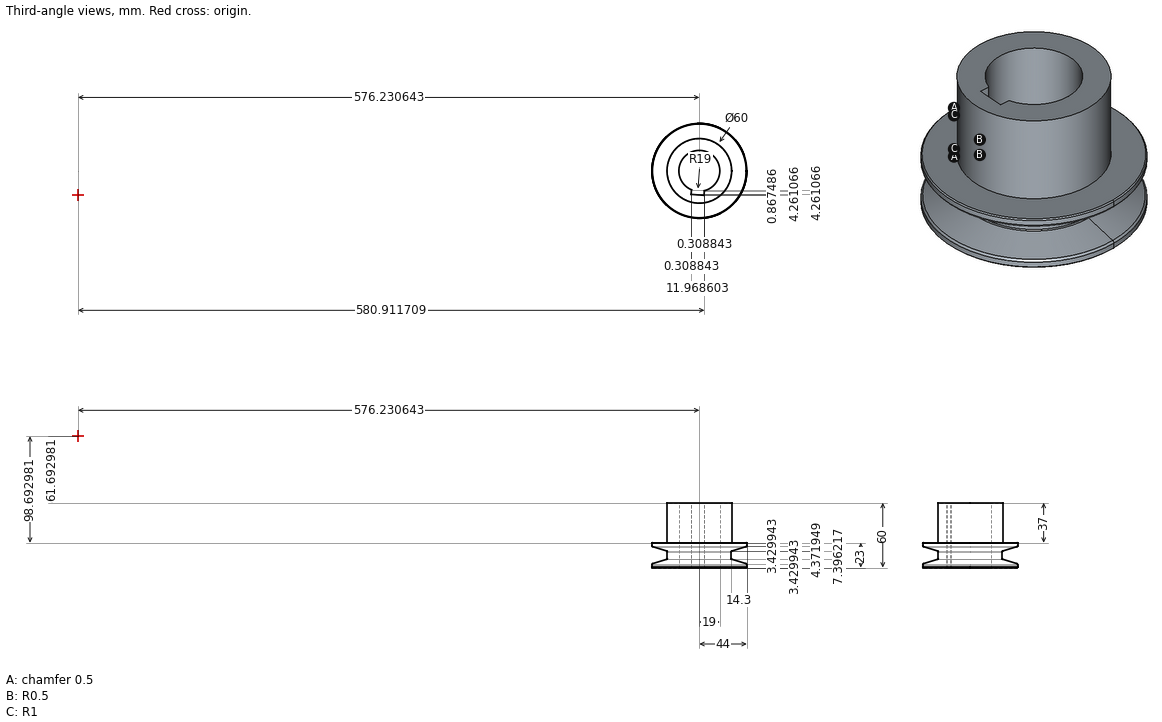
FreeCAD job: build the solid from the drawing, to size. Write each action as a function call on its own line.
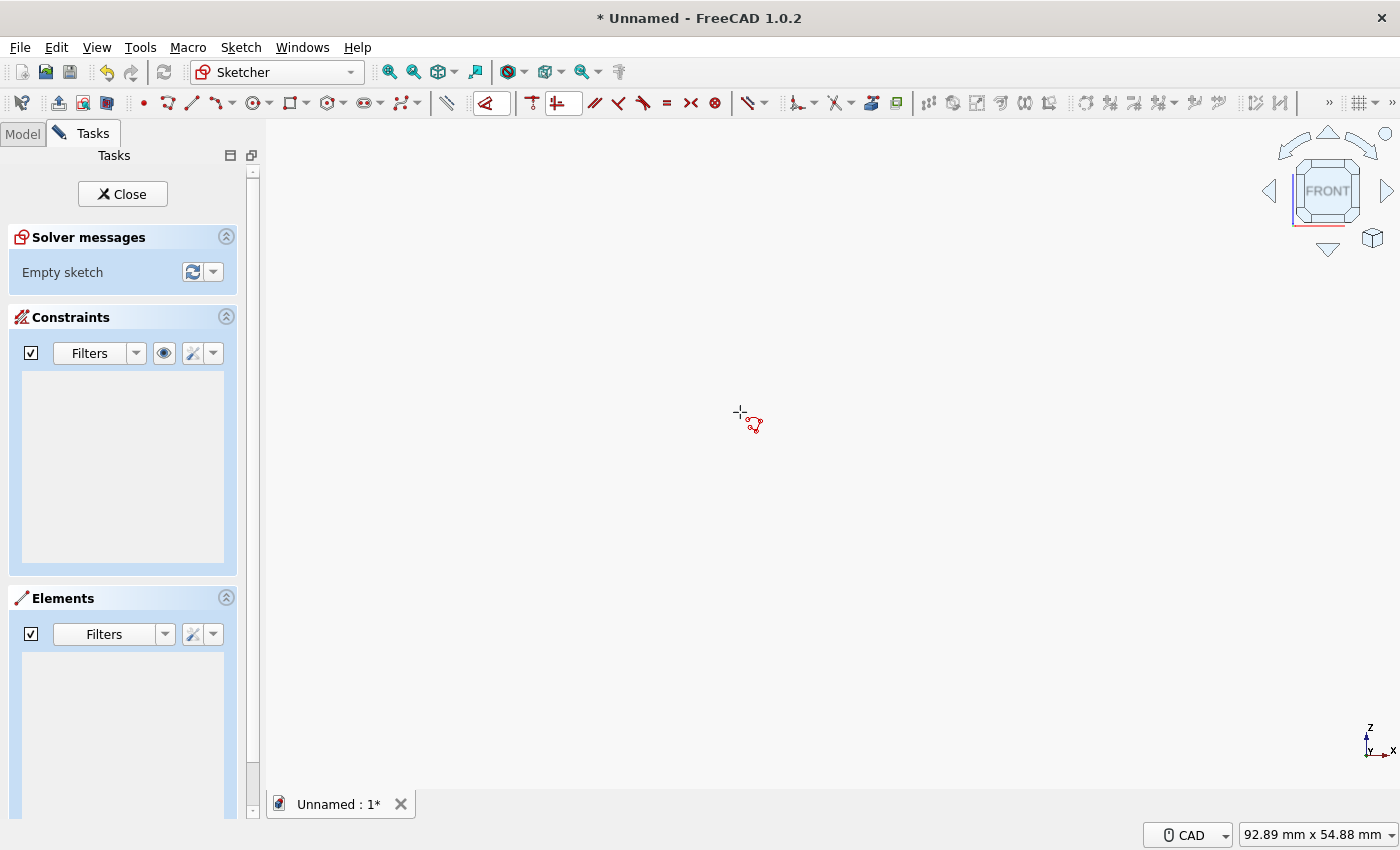
click(495, 370)
click(1032, 370)
click(1032, 411)
click(858, 465)
click(858, 555)
click(1032, 608)
click(1032, 650)
click(495, 650)
click(495, 371)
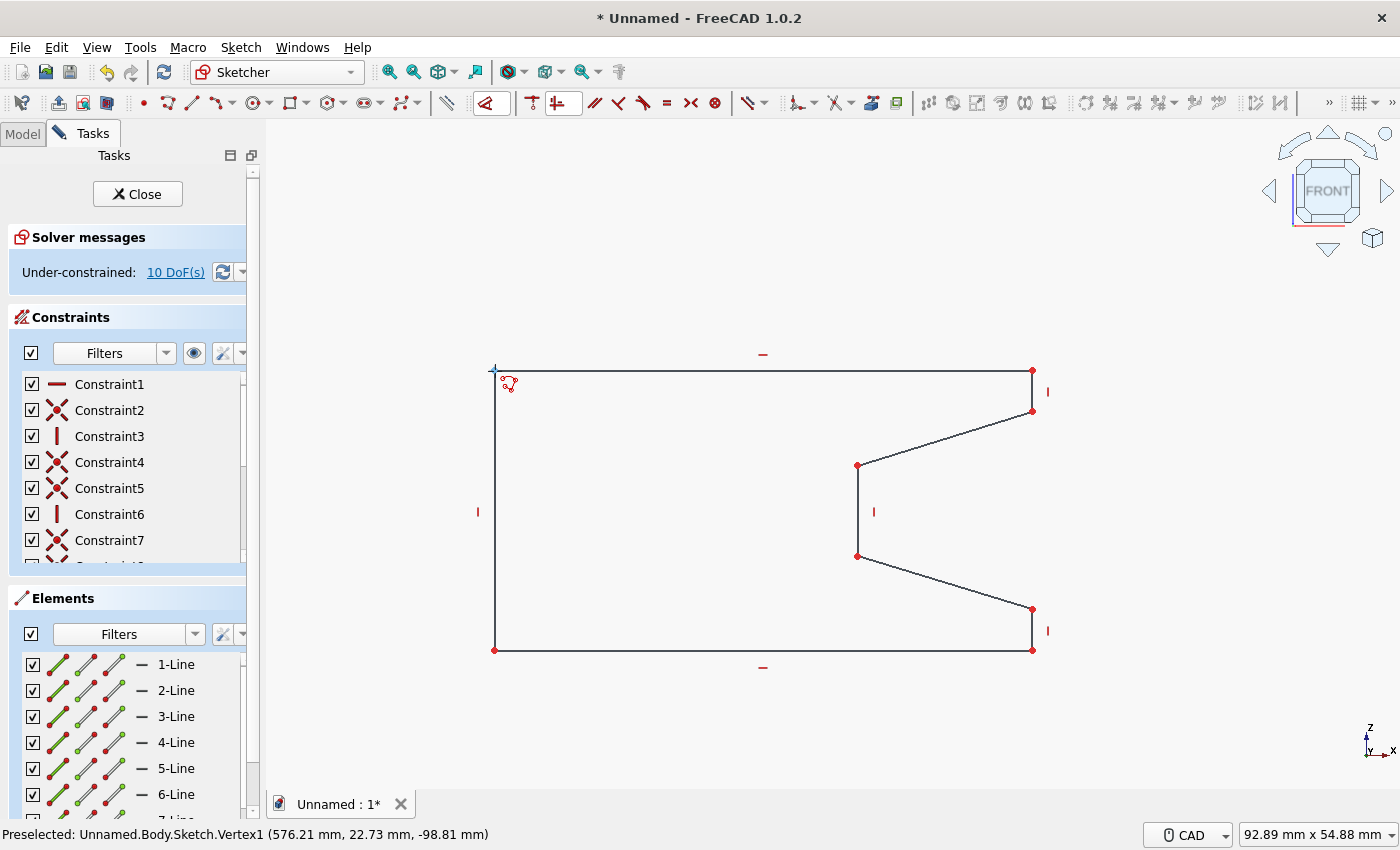
click(192, 104)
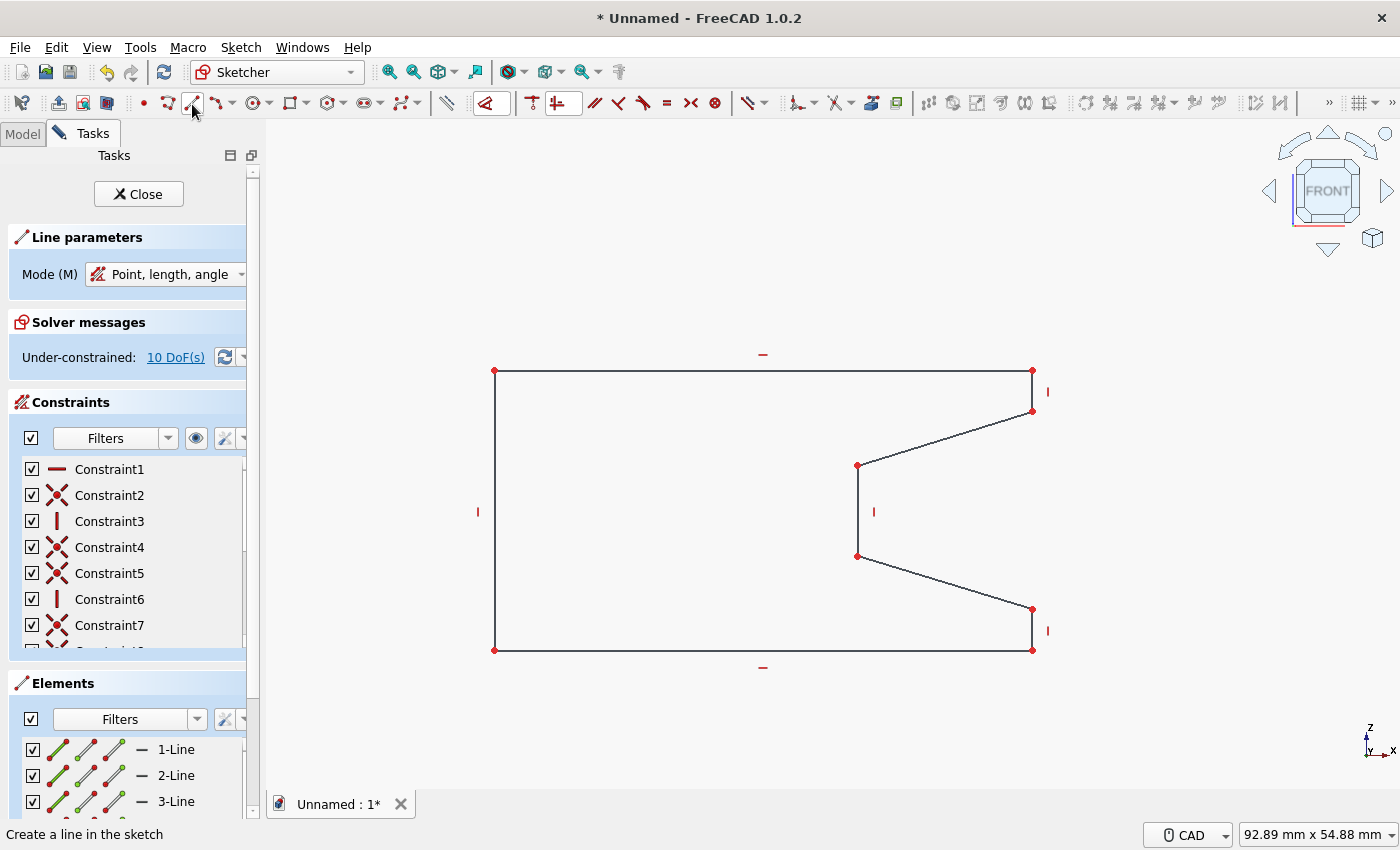
click(495, 341)
click(495, 257)
key(Escape)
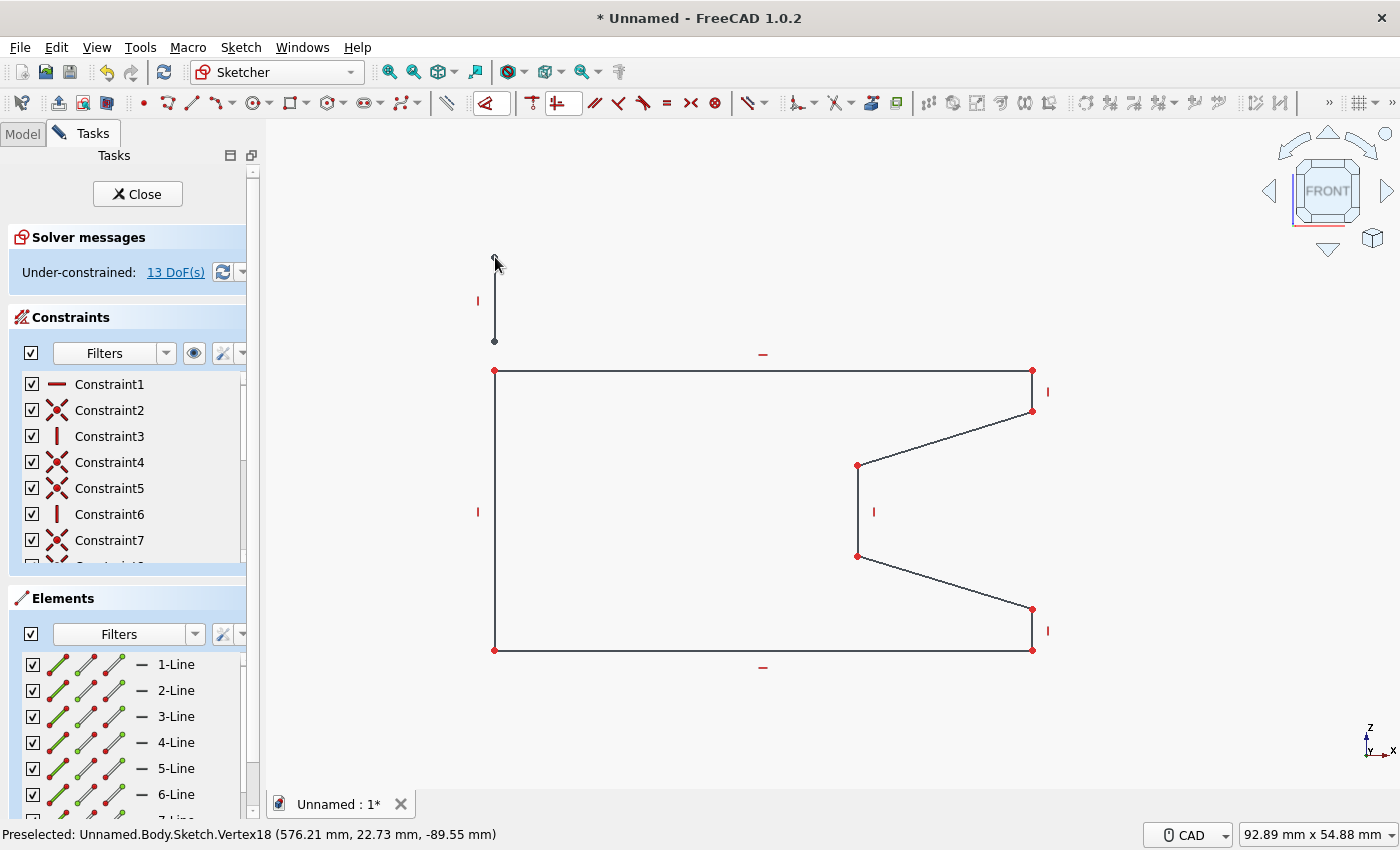
click(495, 317)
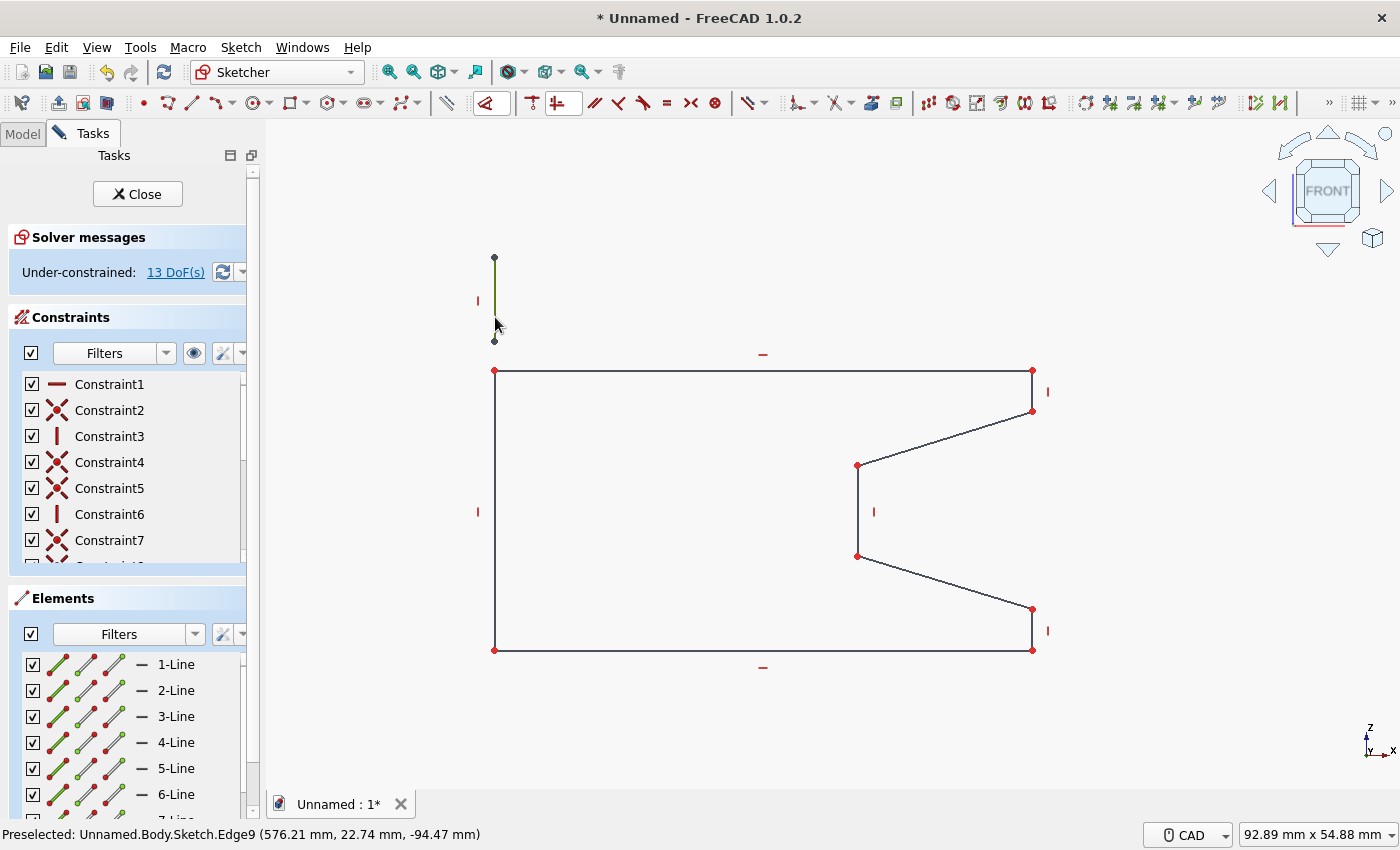
click(448, 104)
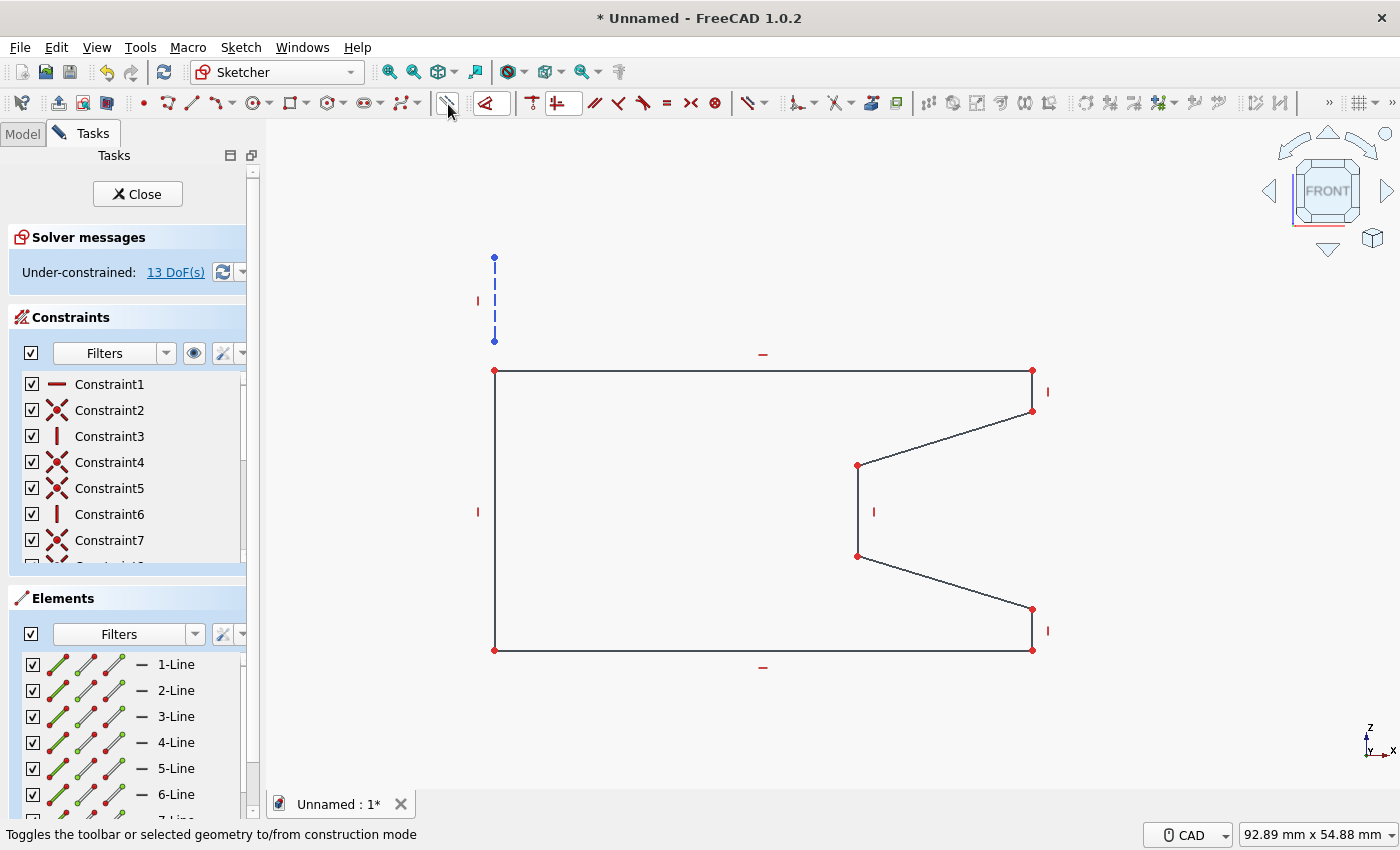
click(486, 104)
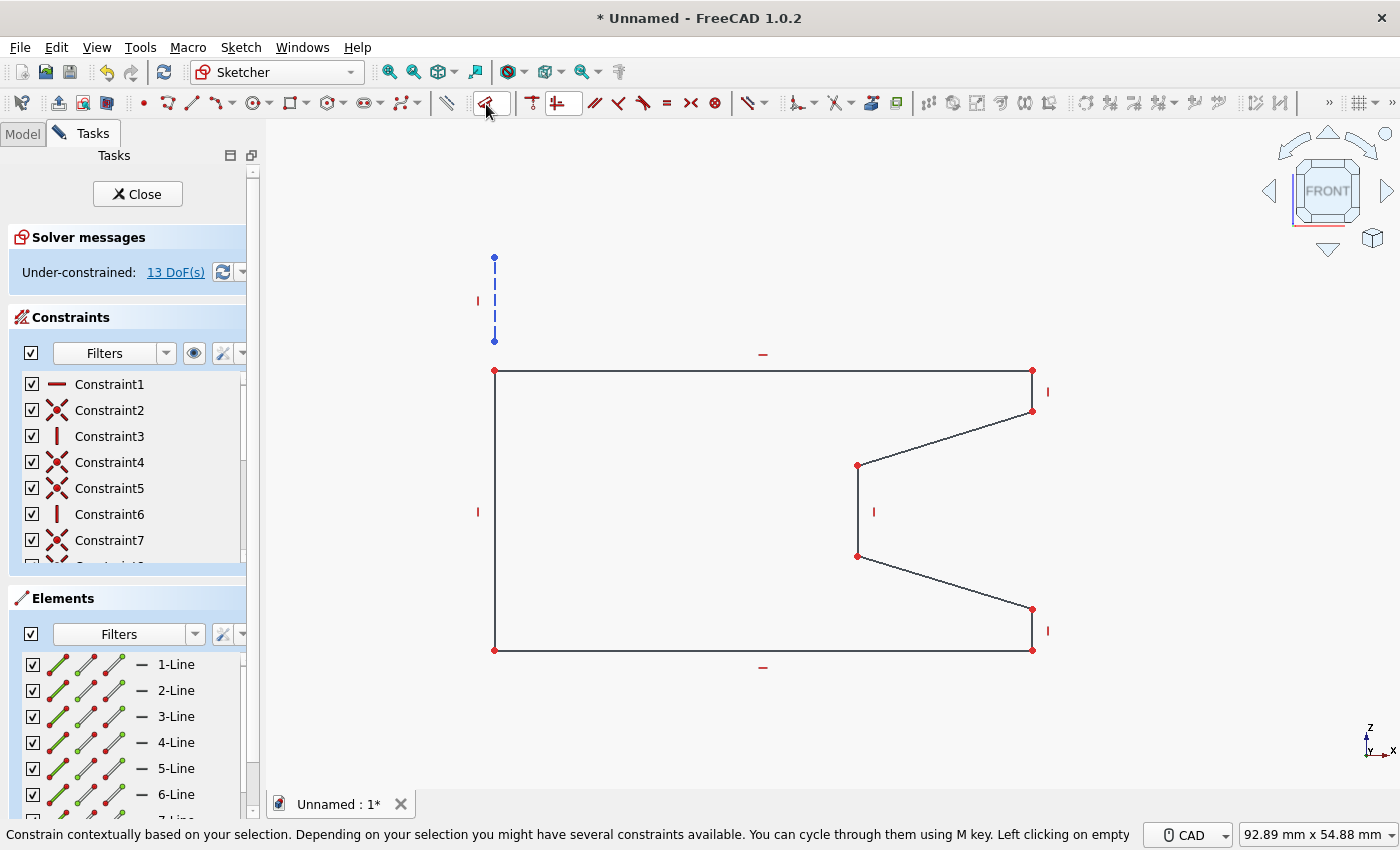
click(656, 371)
click(763, 337)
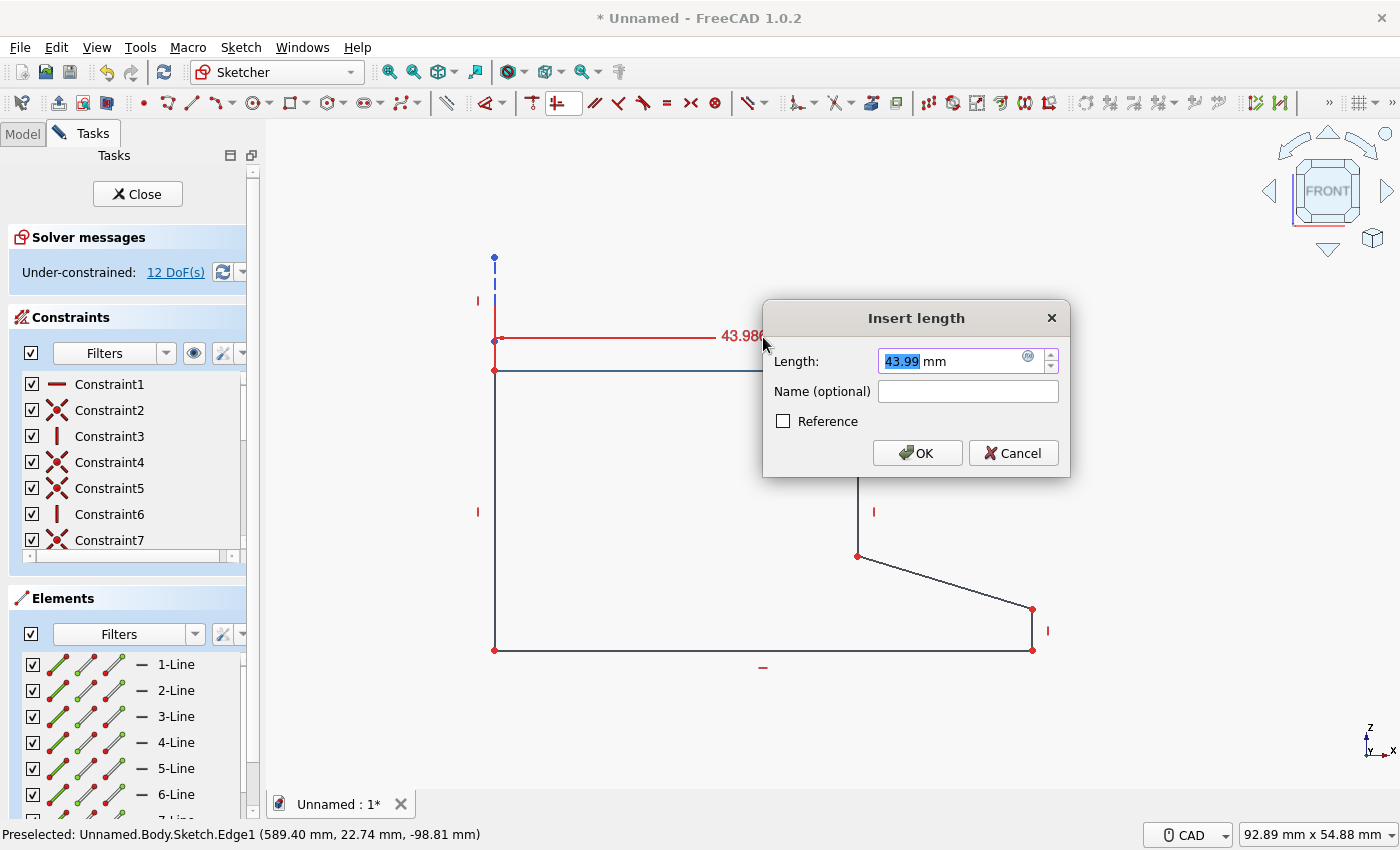
text(44)
key(Return)